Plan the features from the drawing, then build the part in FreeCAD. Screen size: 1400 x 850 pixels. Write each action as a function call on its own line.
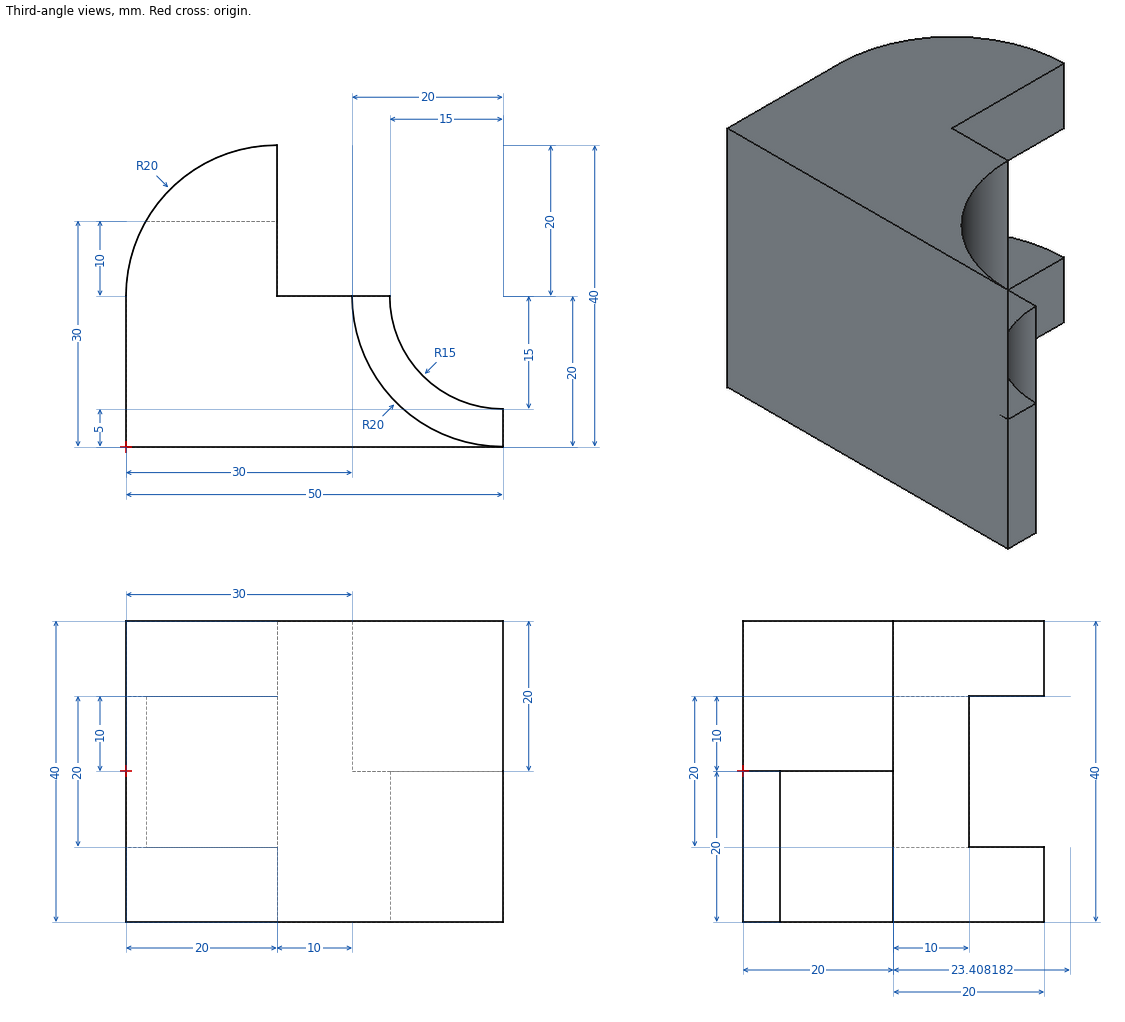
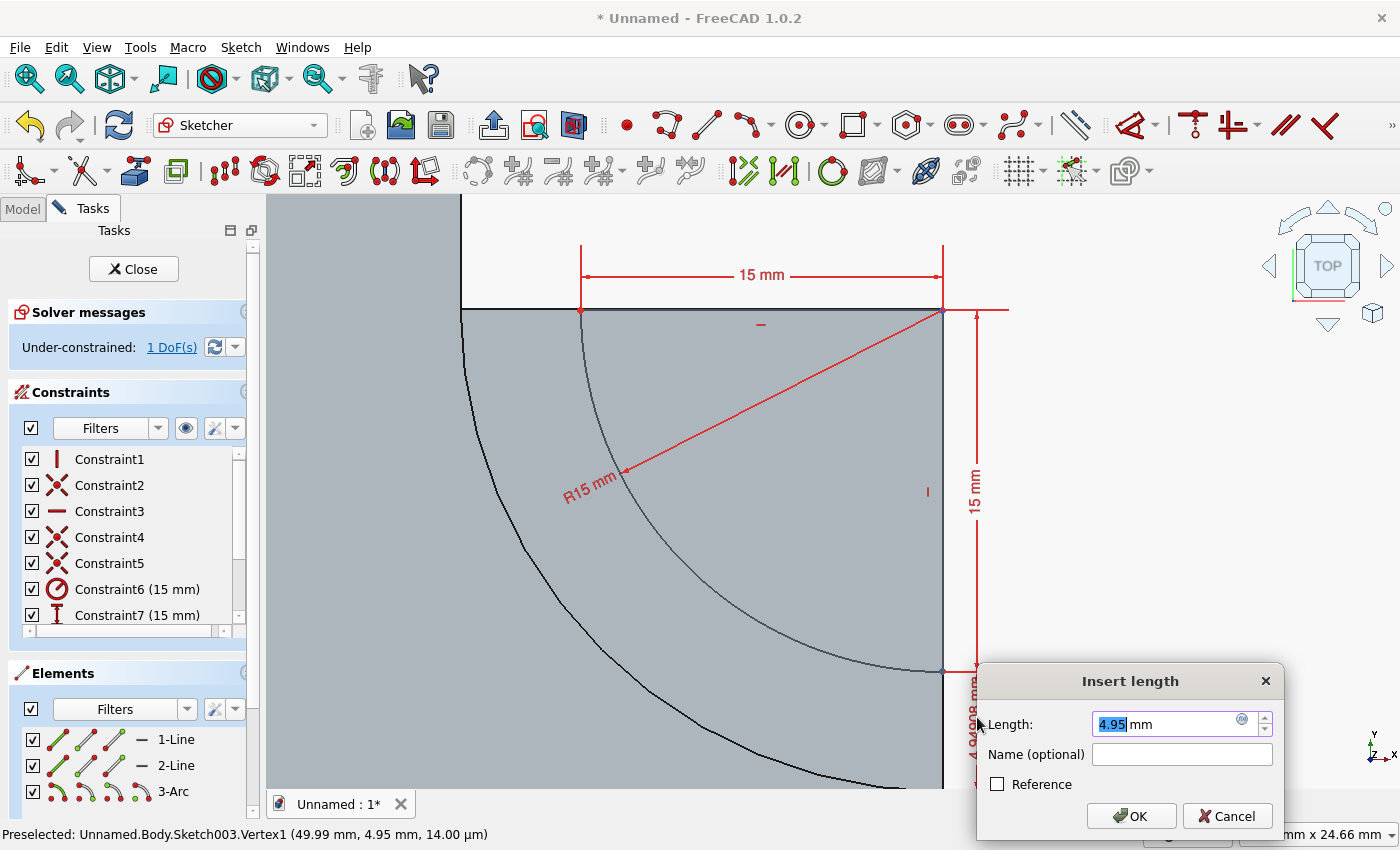
text(5)
key(Return)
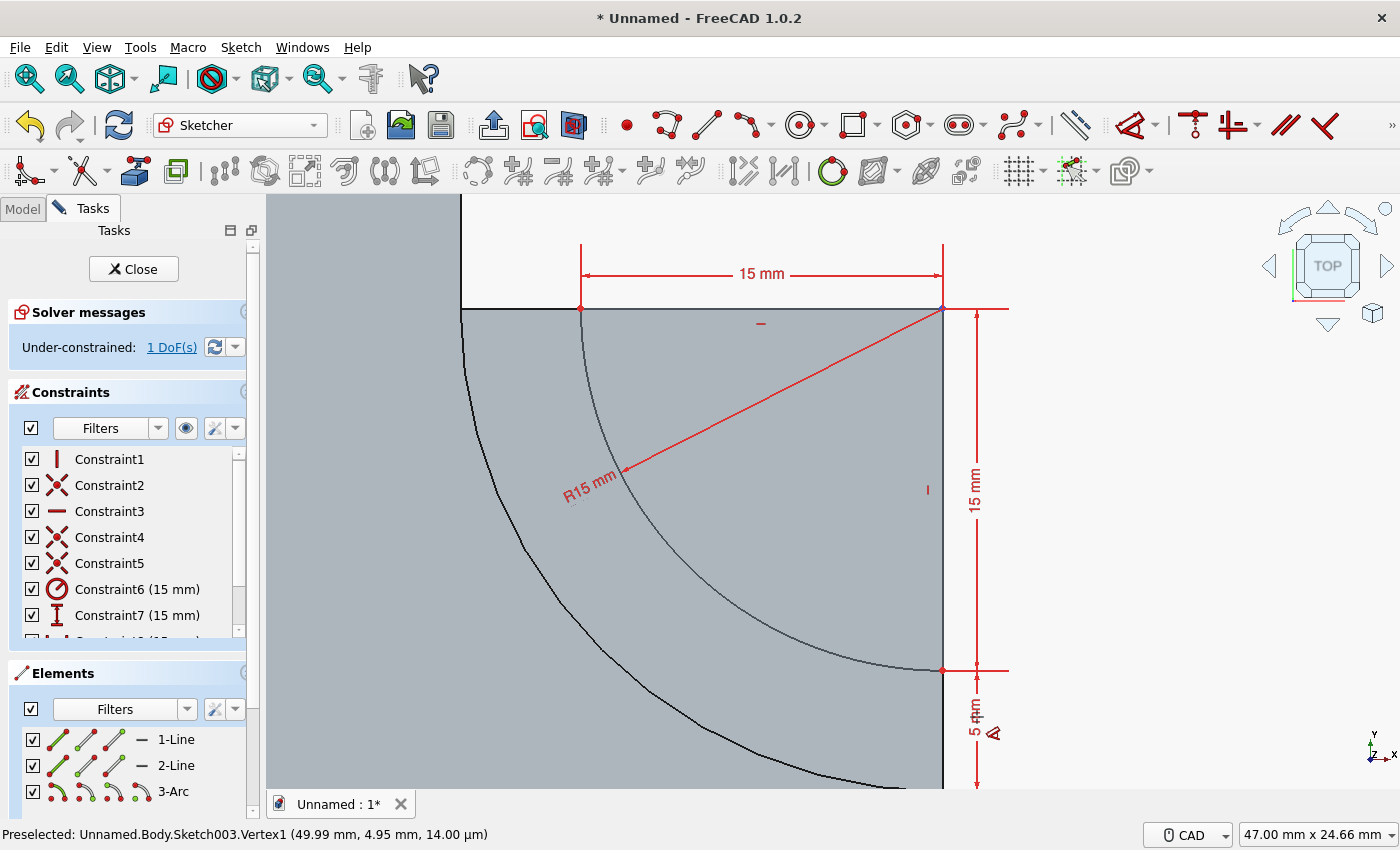
click(943, 671)
click(618, 637)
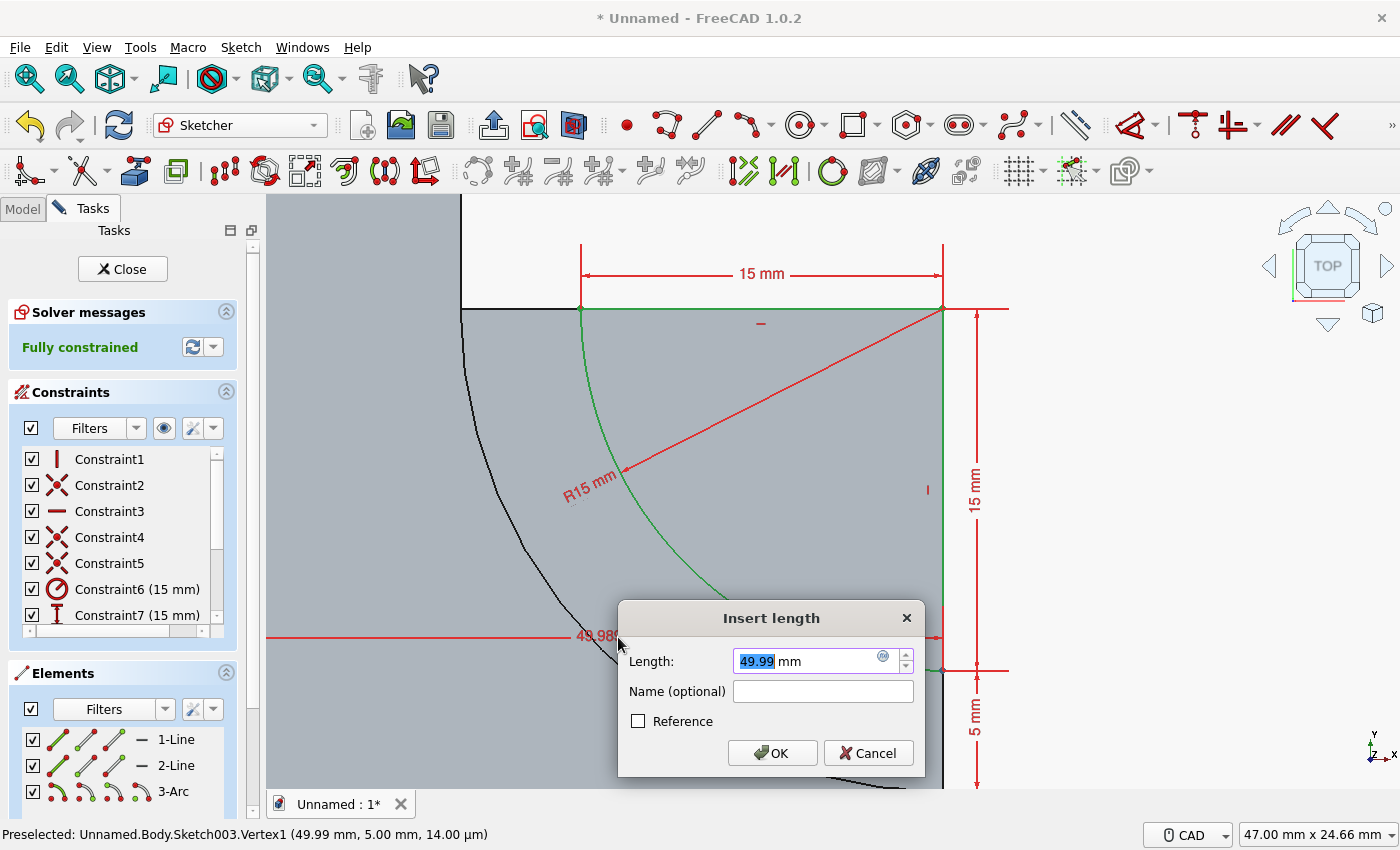
text(50)
key(Return)
key(Escape)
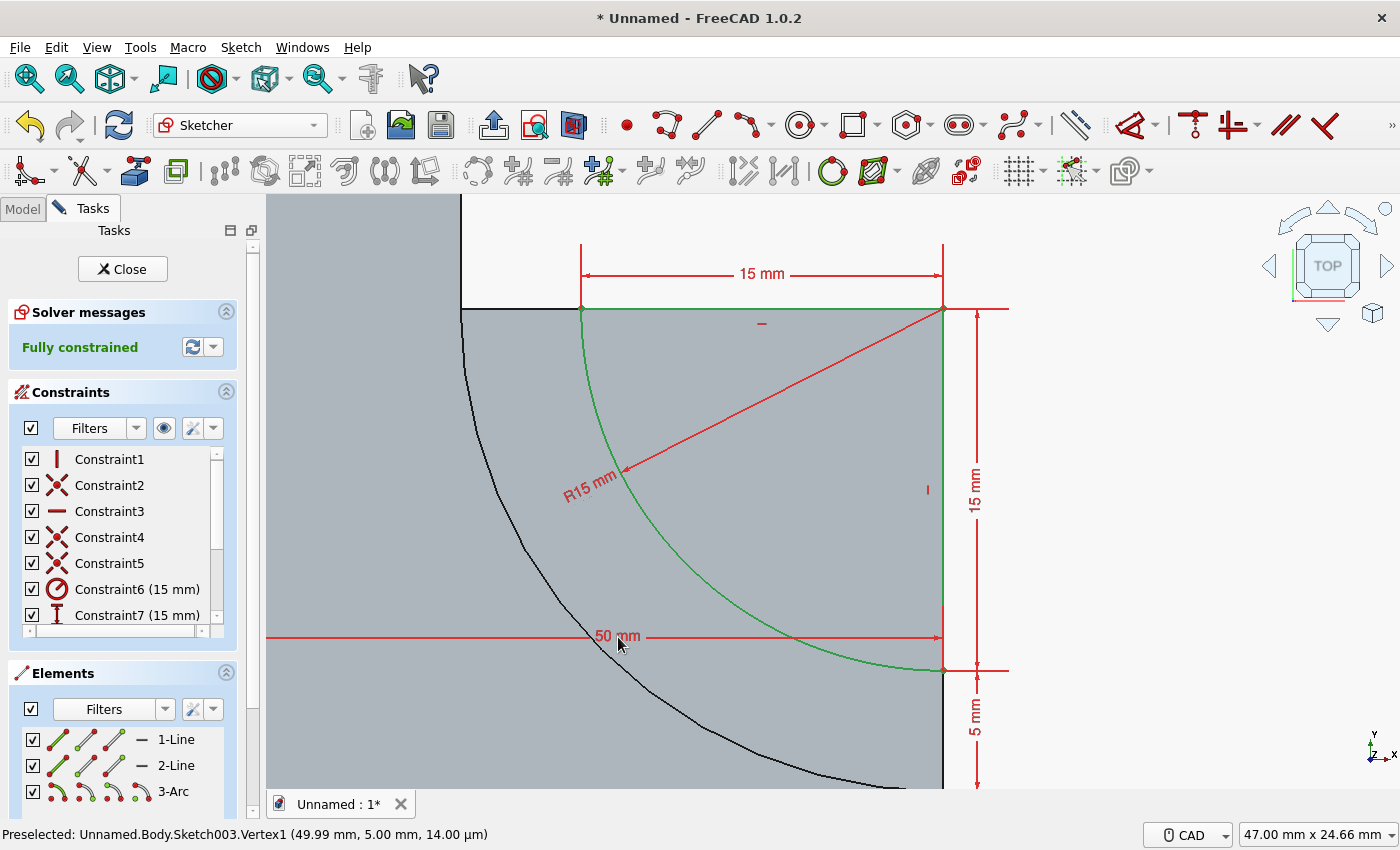
click(123, 269)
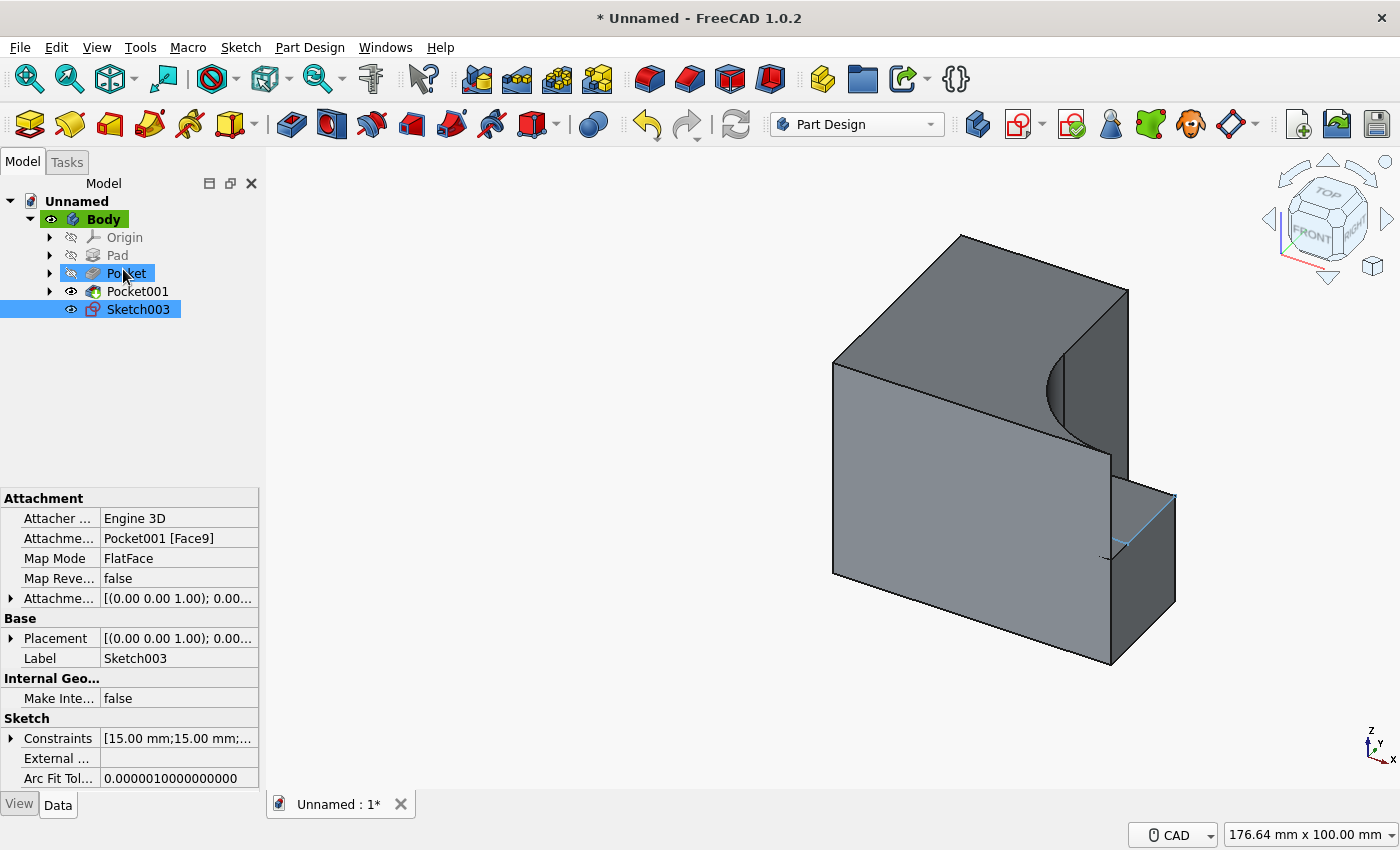
click(292, 124)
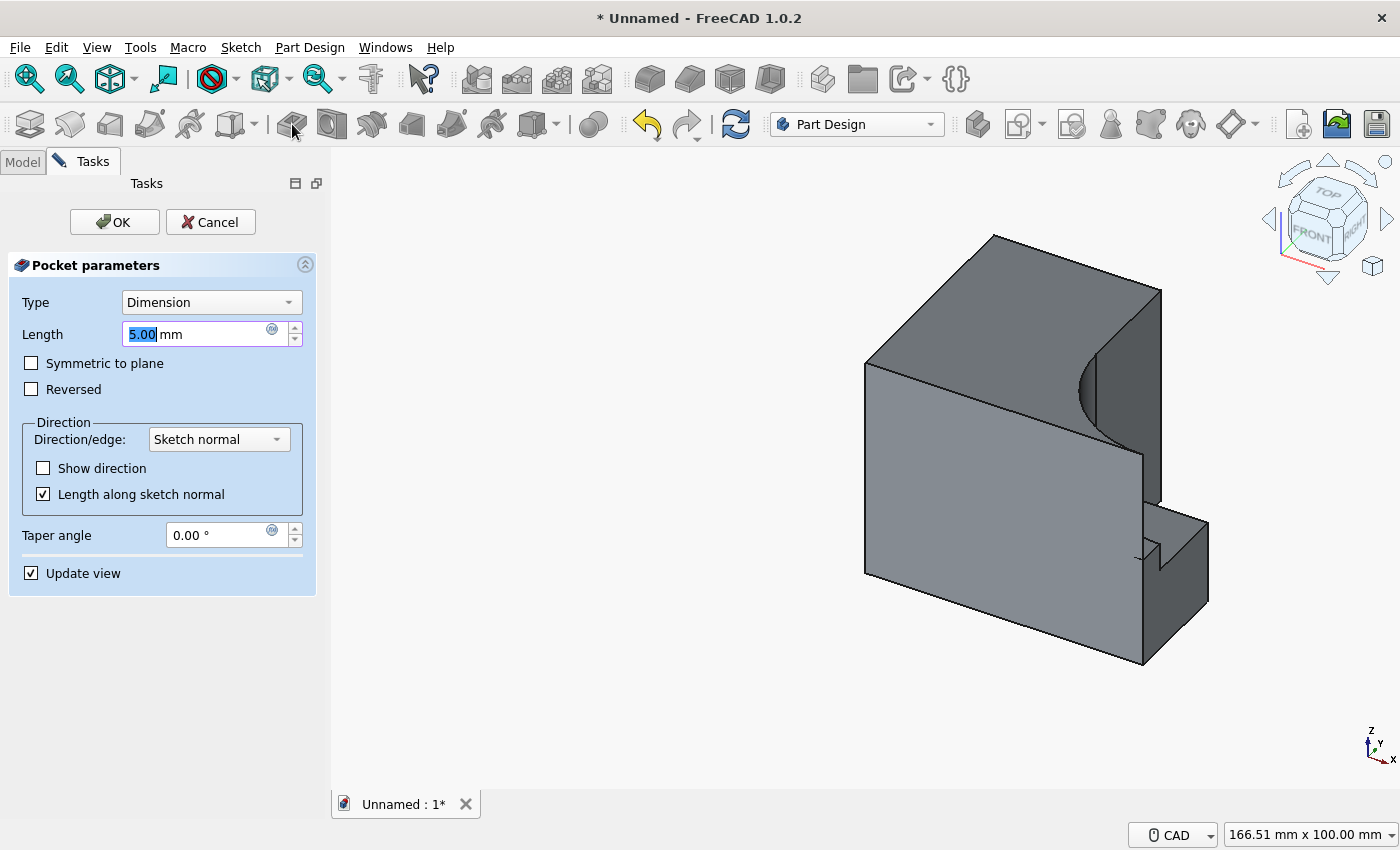
text(20)
key(Tab)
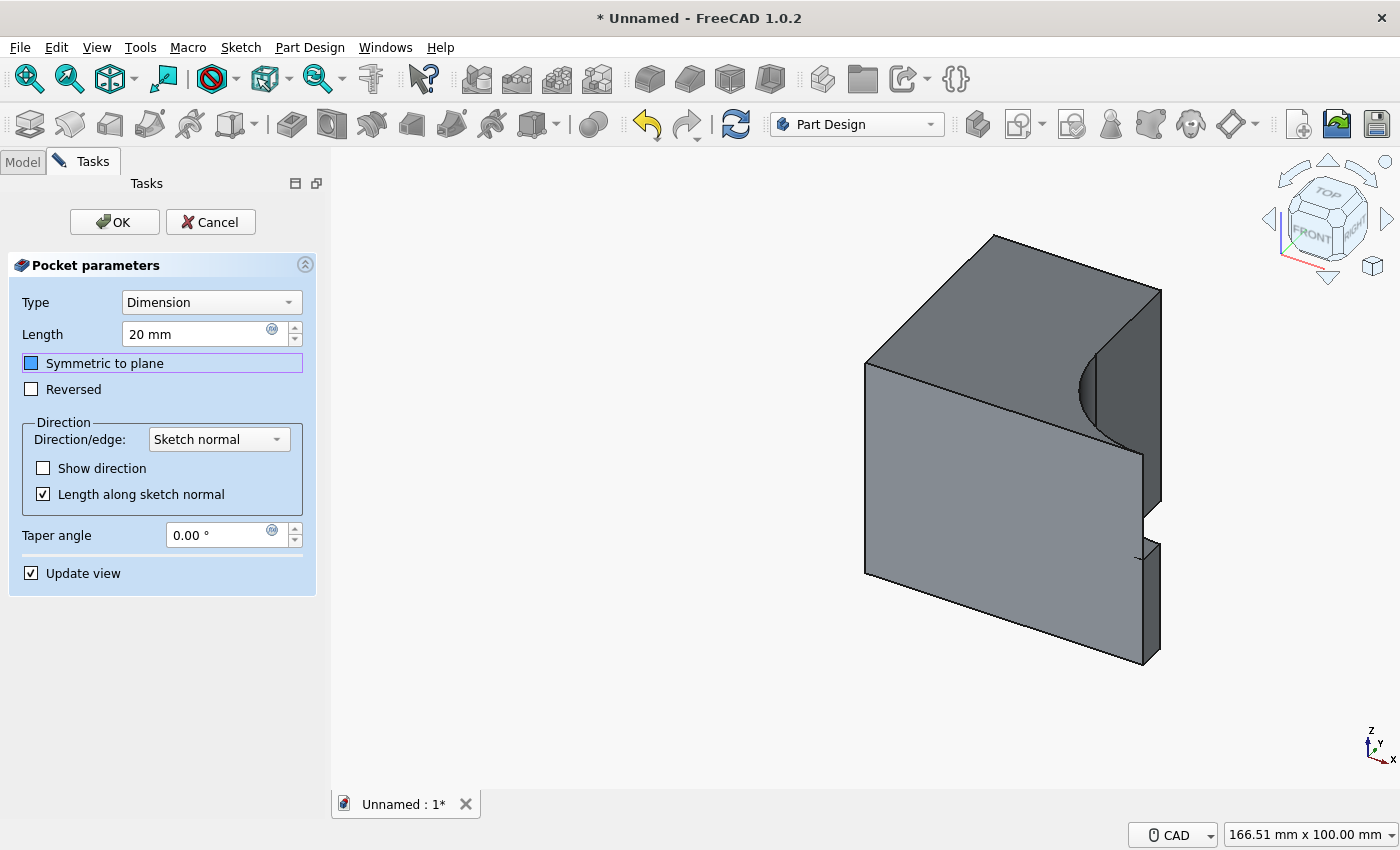
click(115, 222)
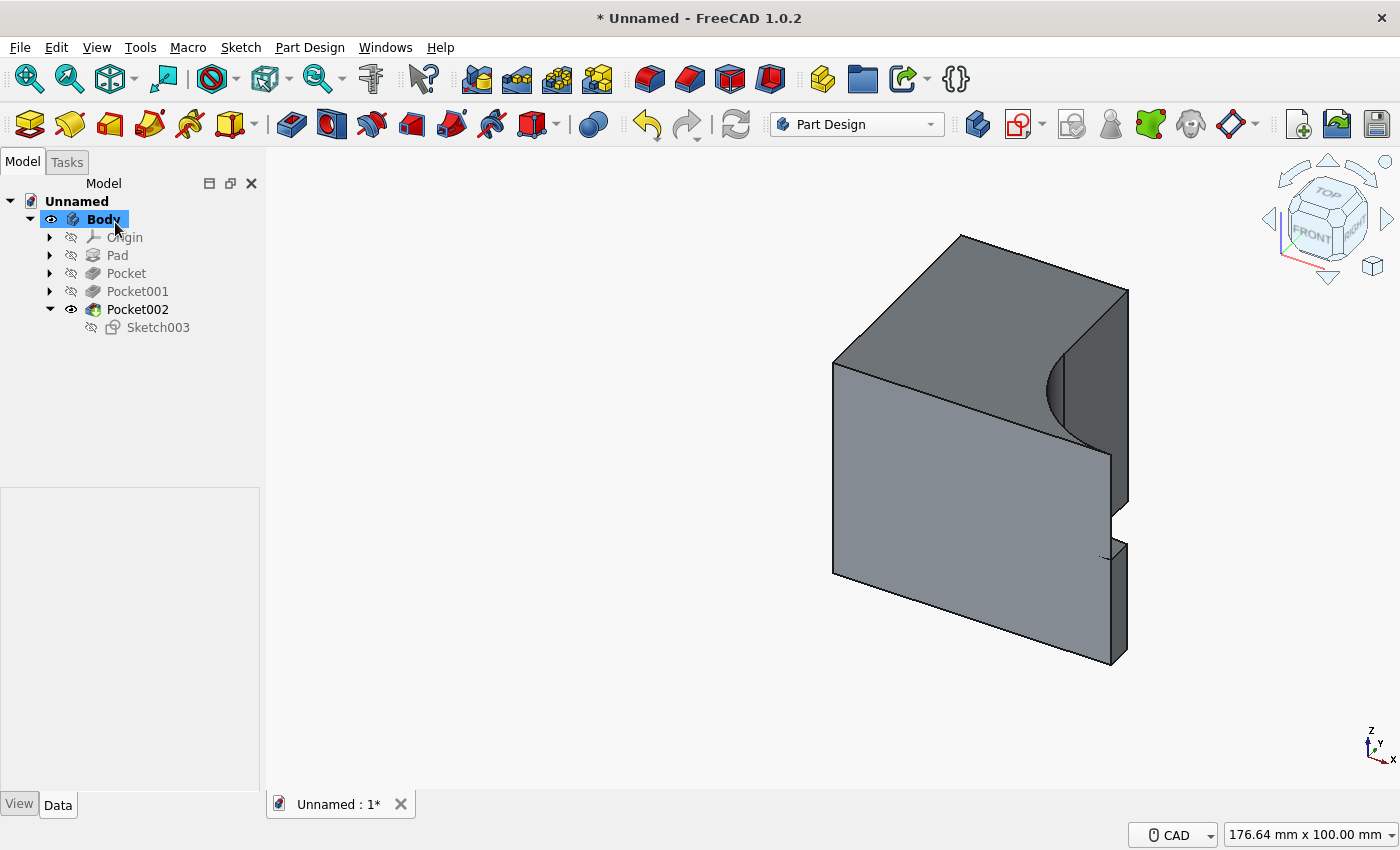
click(978, 349)